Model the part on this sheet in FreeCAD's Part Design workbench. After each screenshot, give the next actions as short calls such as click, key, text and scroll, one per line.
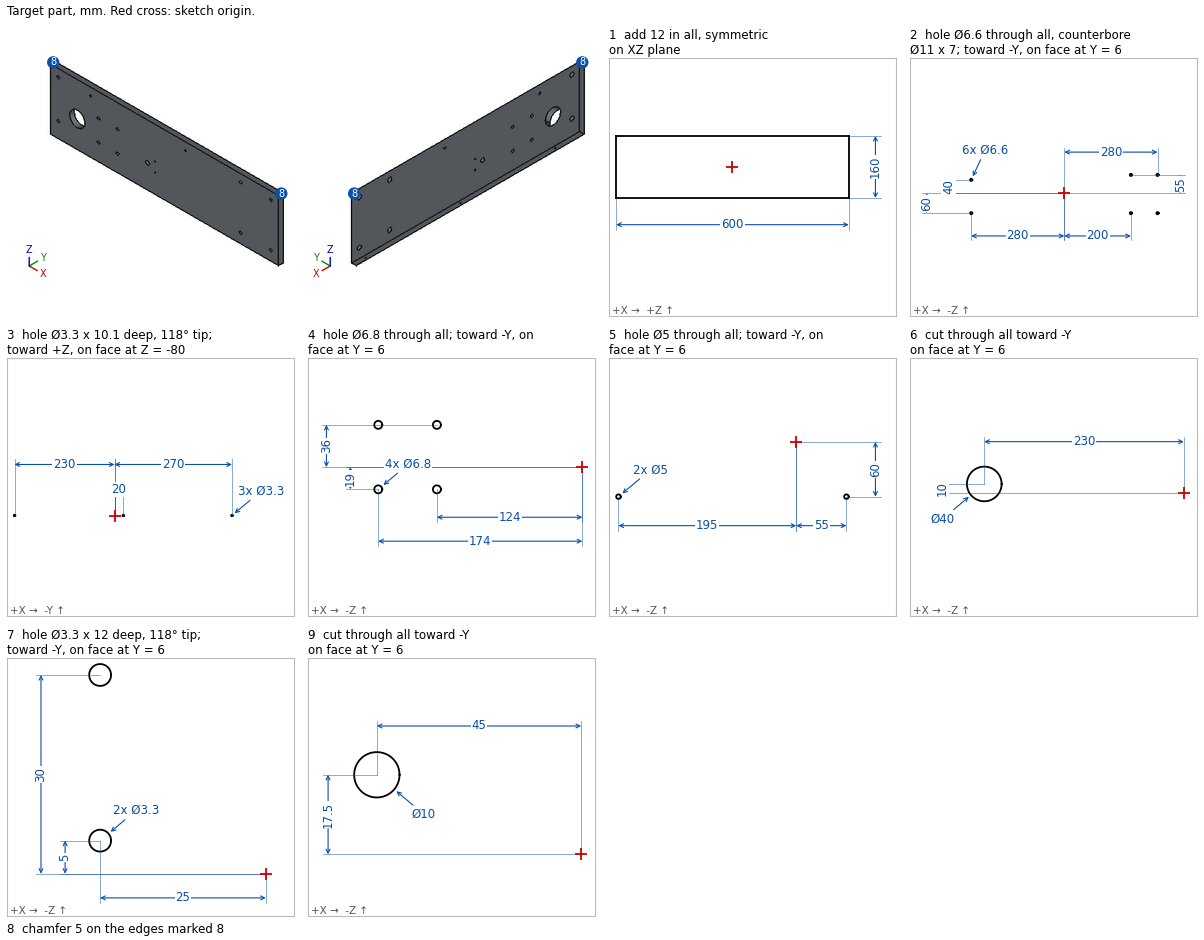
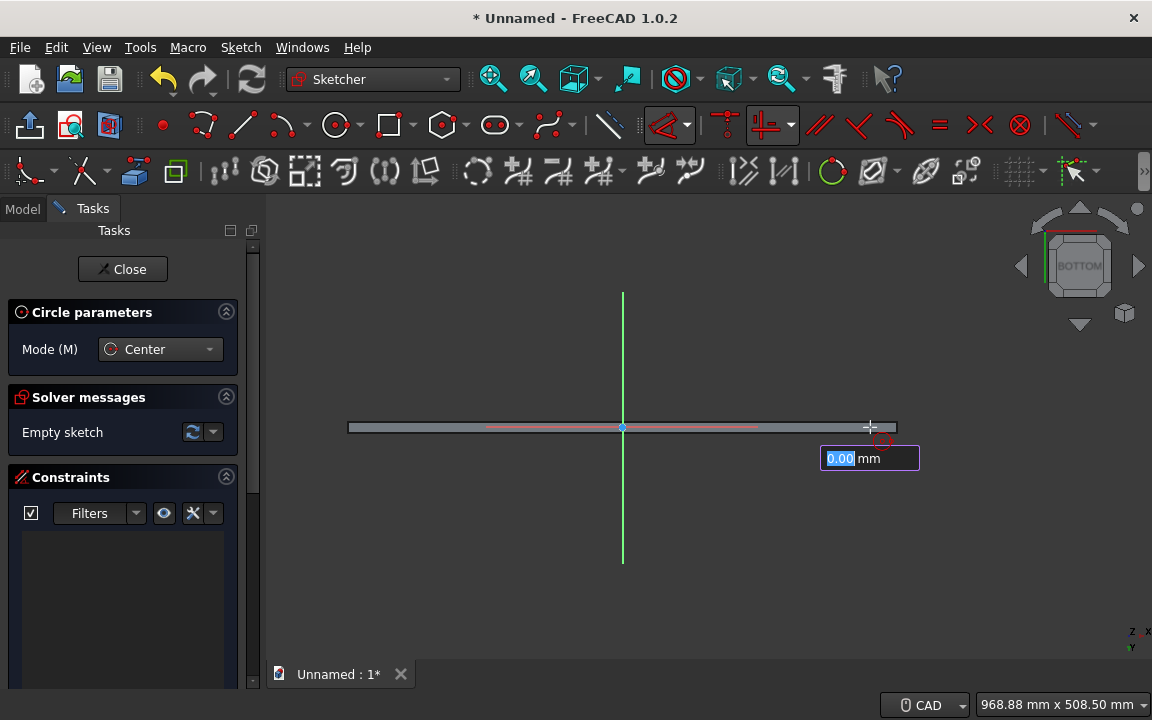
scroll(870, 426, up, 13)
move(862, 420)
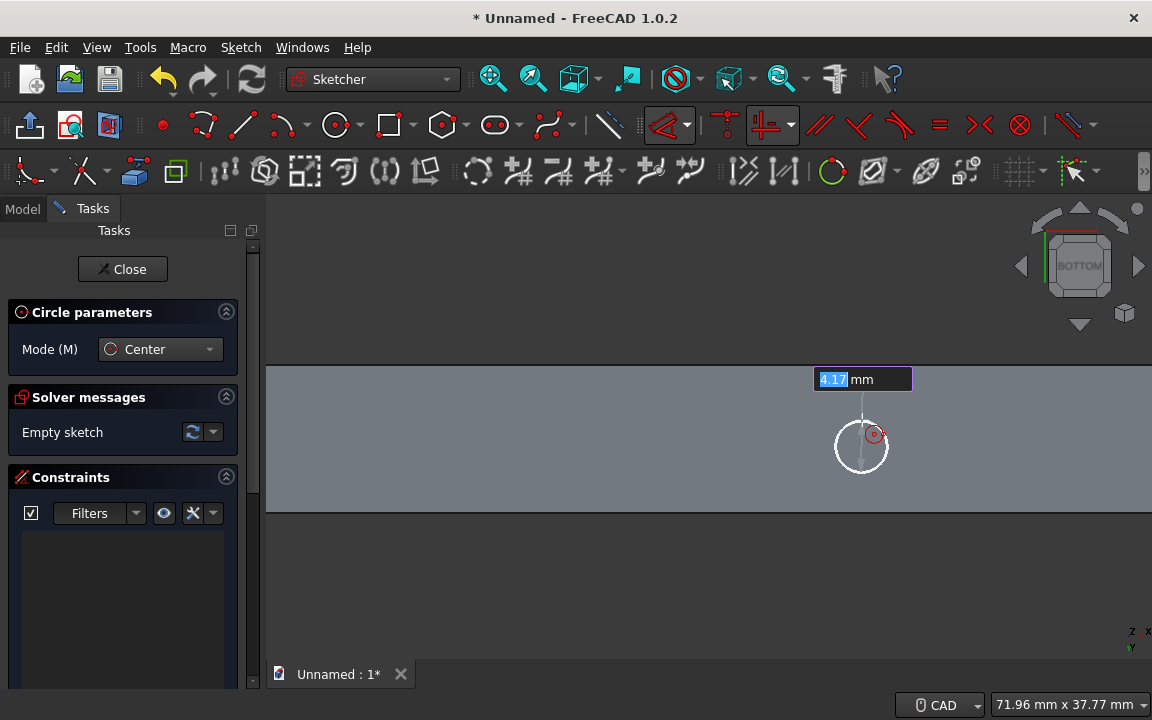
text(3.3)
key(Return)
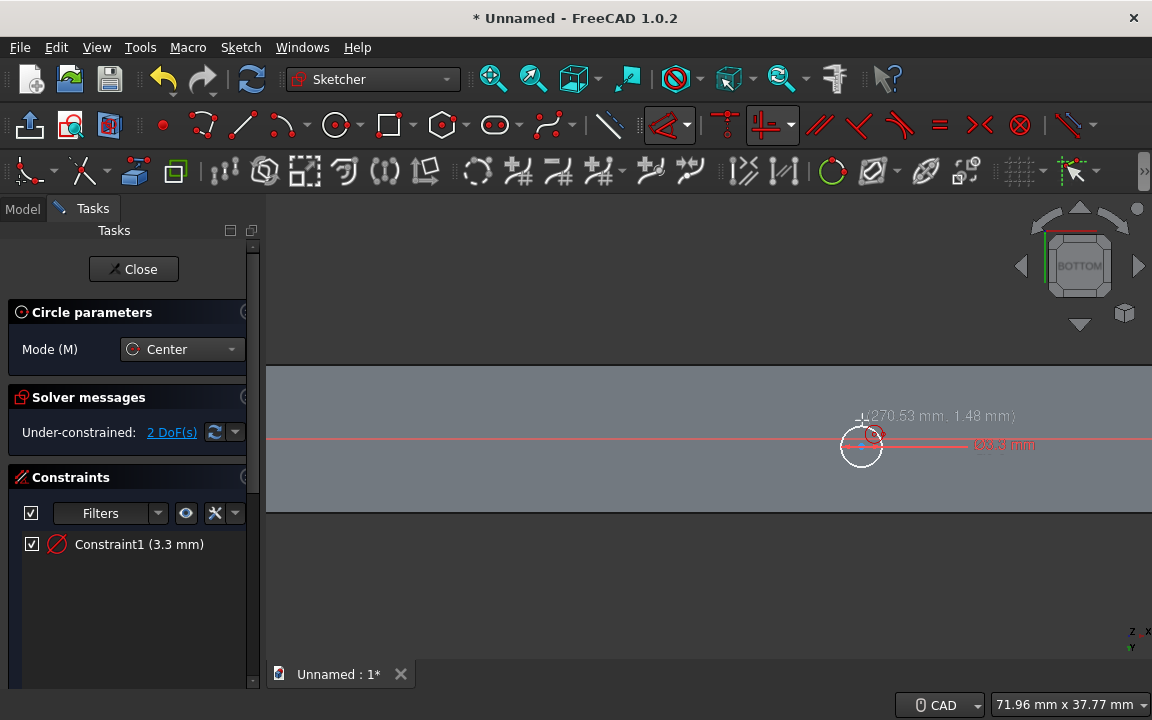
scroll(870, 425, down, 13)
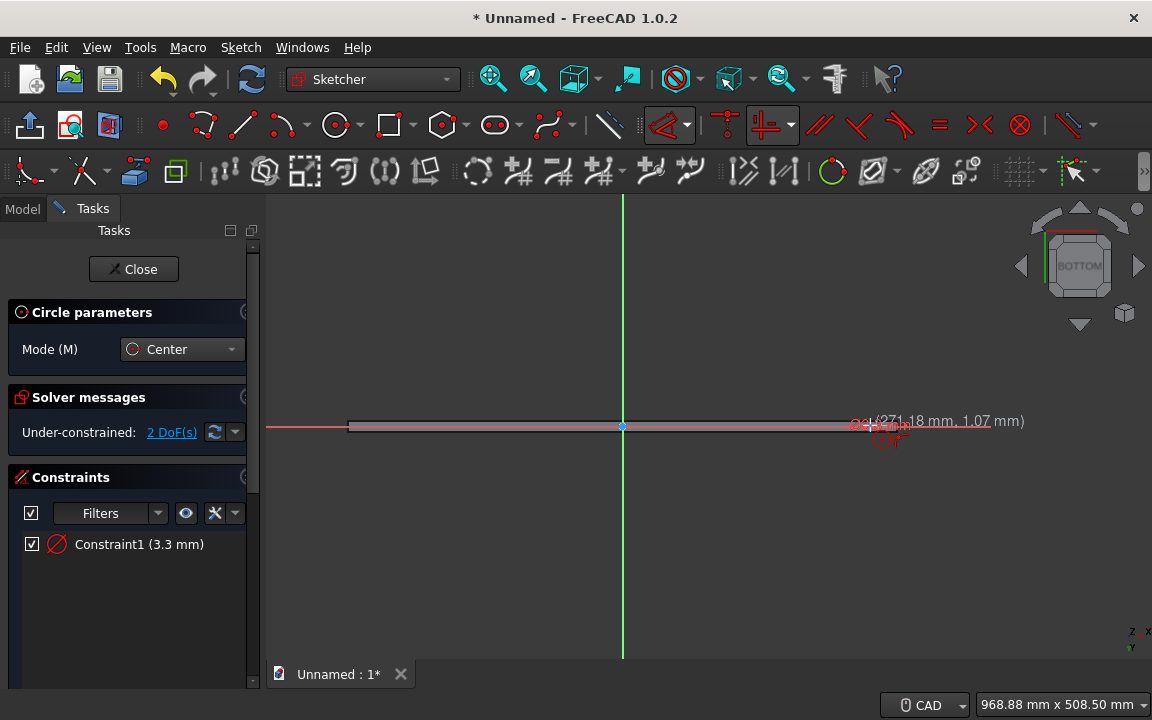
scroll(641, 427, up, 14)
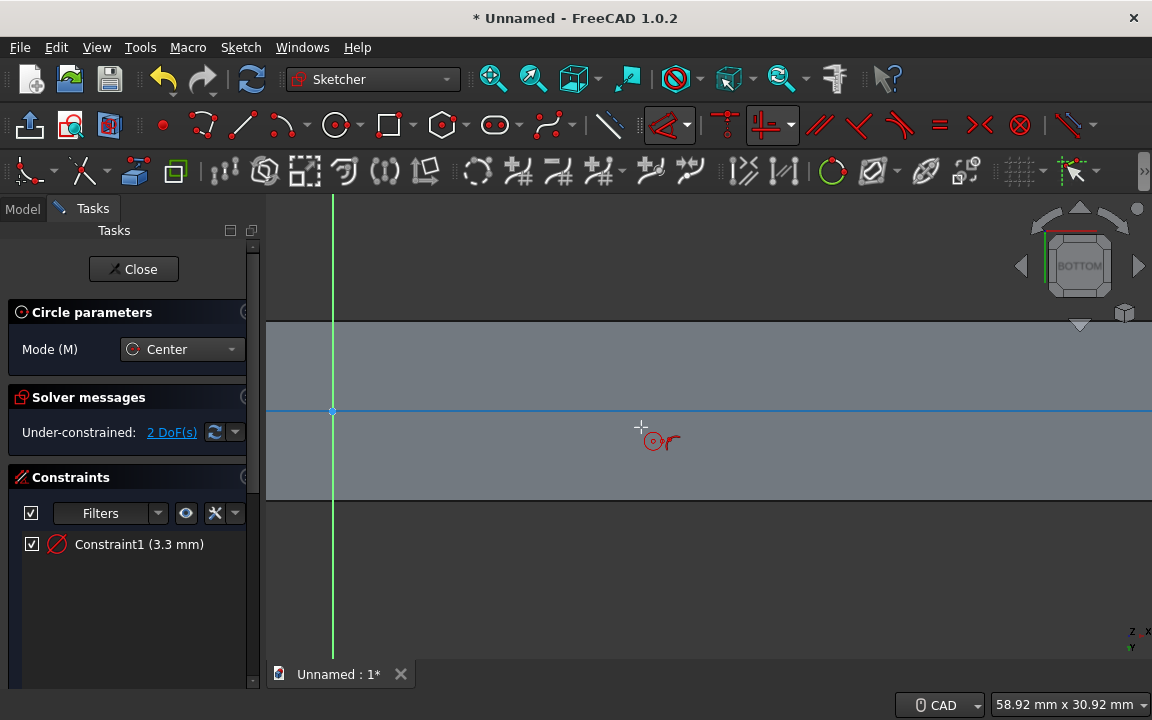
scroll(641, 427, down, 14)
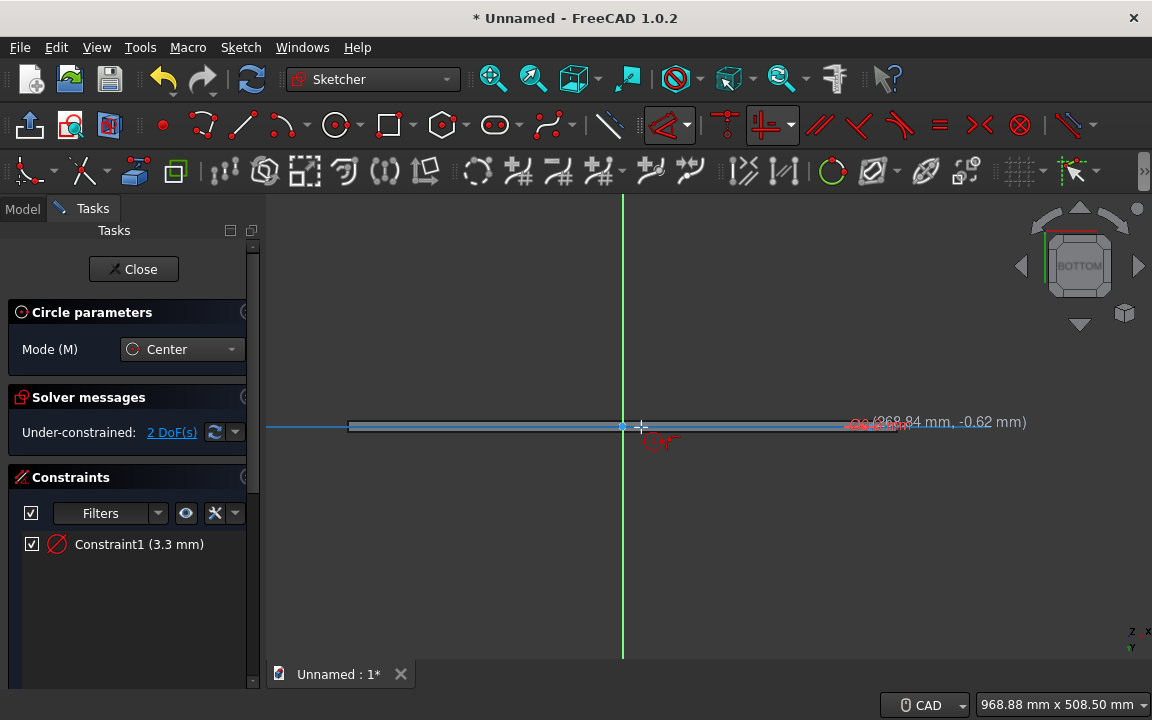
click(641, 427)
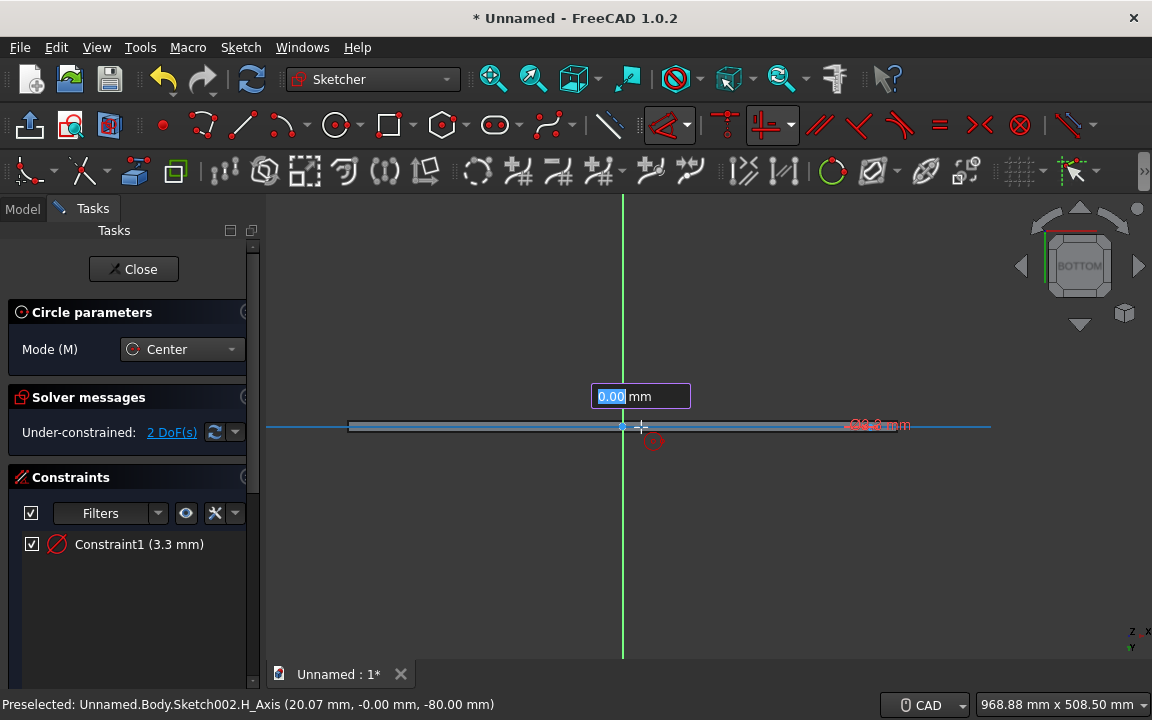
scroll(641, 425, up, 13)
move(642, 420)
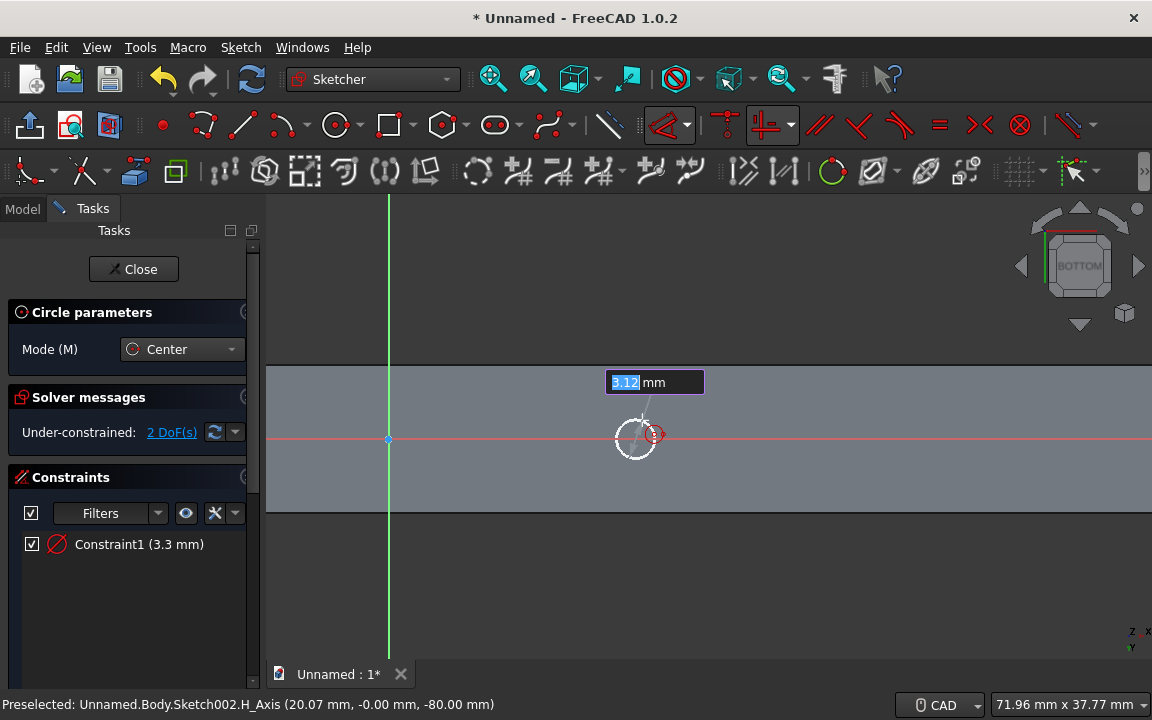
text(3.3)
key(Return)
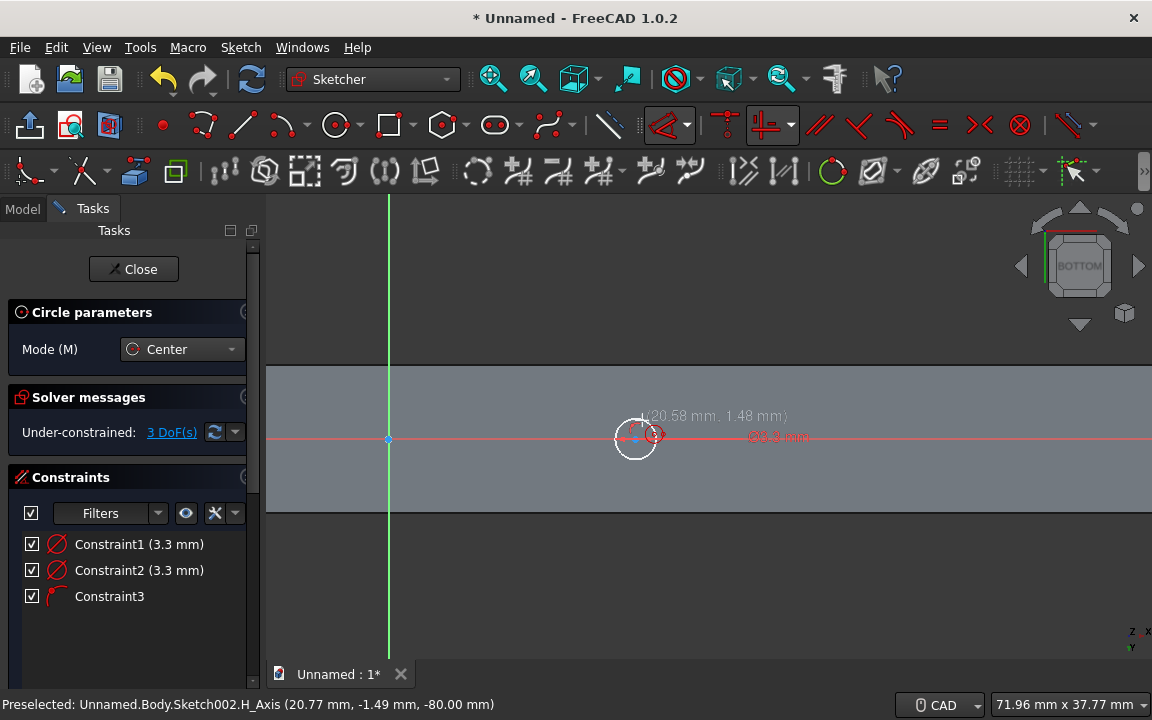
scroll(641, 425, down, 13)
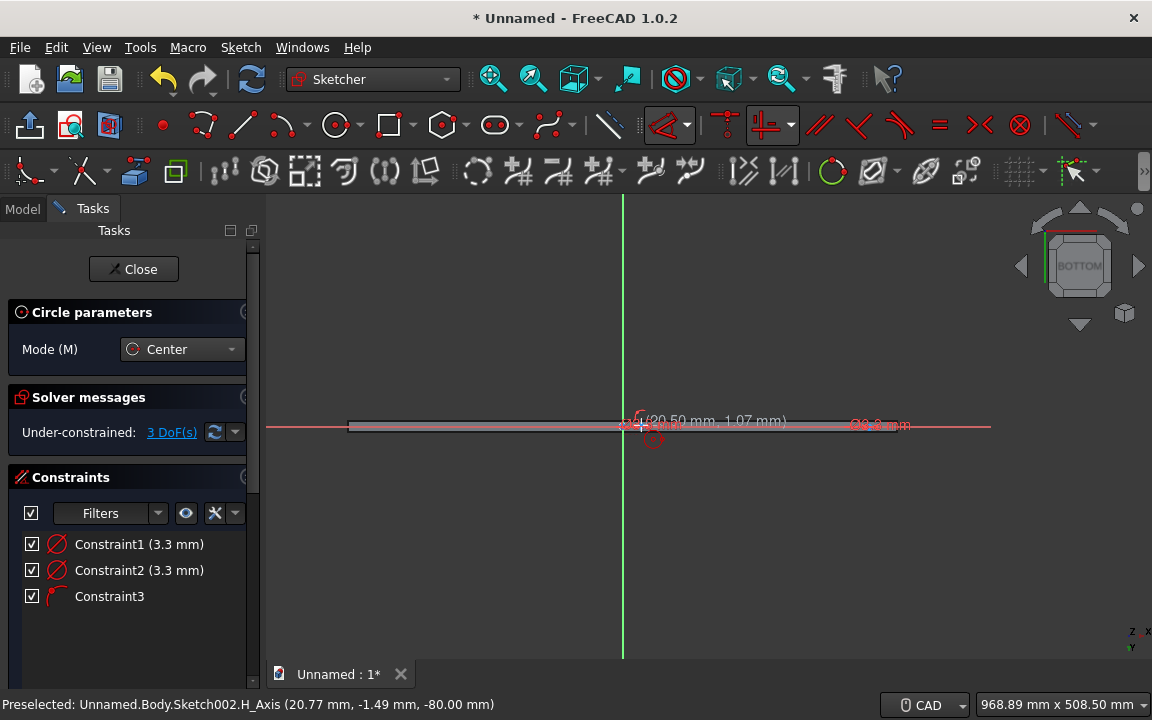
scroll(412, 427, up, 14)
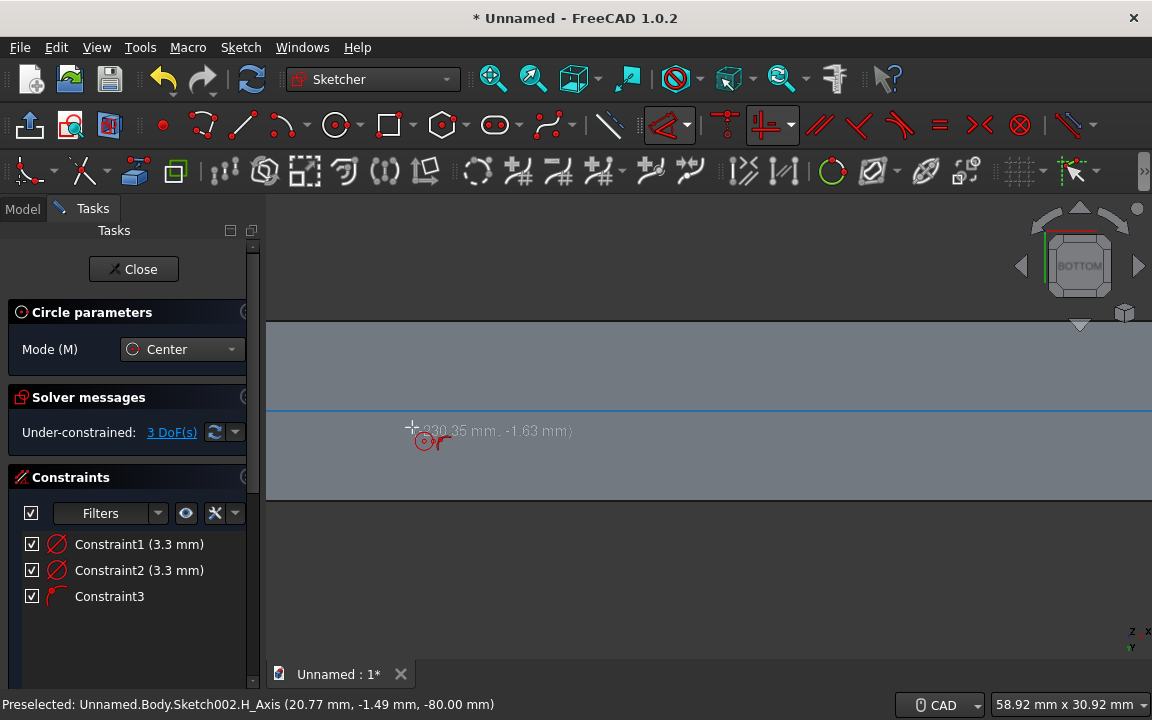
scroll(412, 427, down, 14)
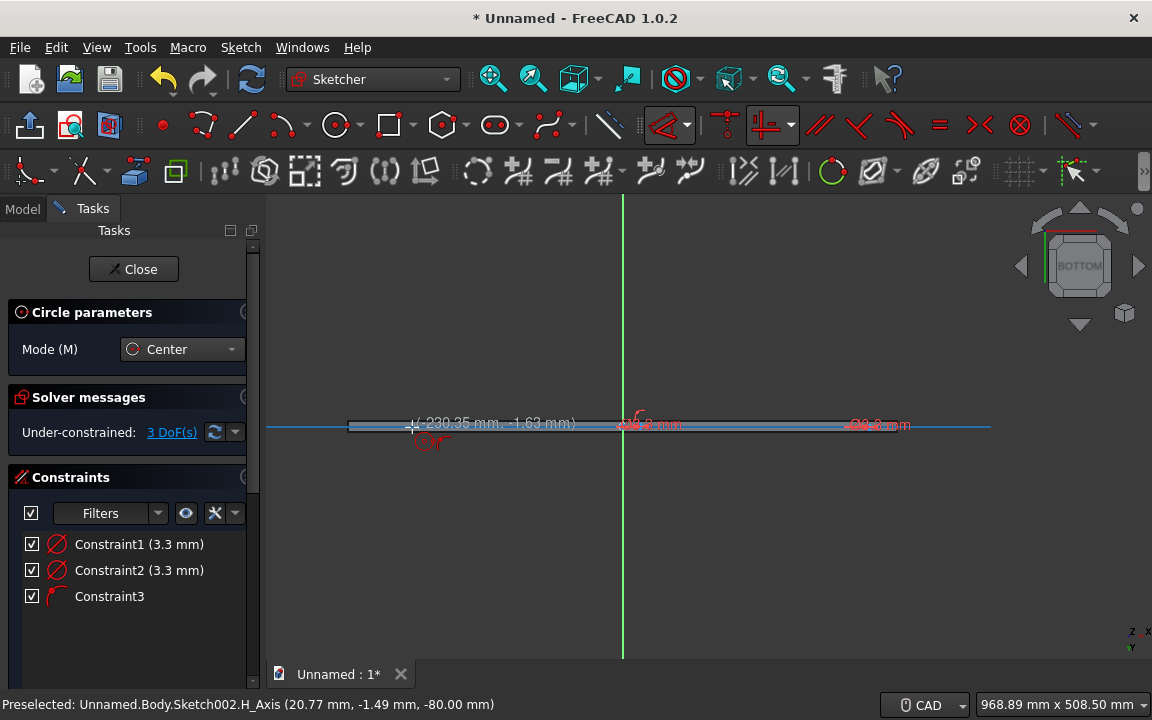
click(412, 427)